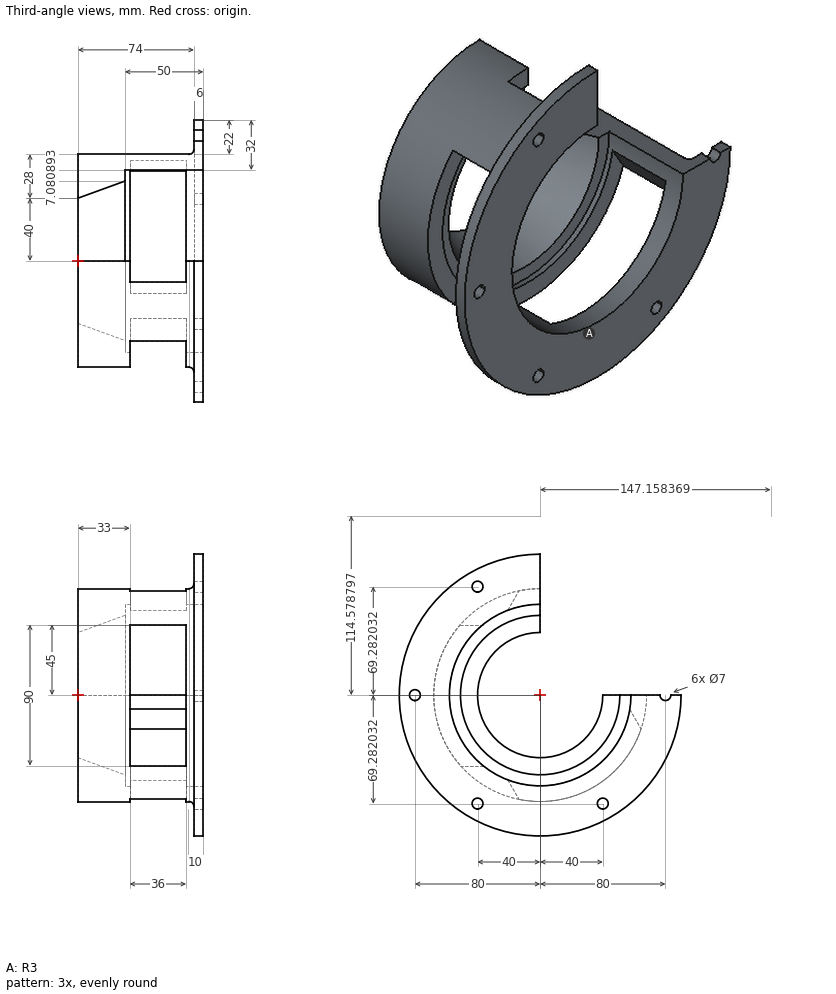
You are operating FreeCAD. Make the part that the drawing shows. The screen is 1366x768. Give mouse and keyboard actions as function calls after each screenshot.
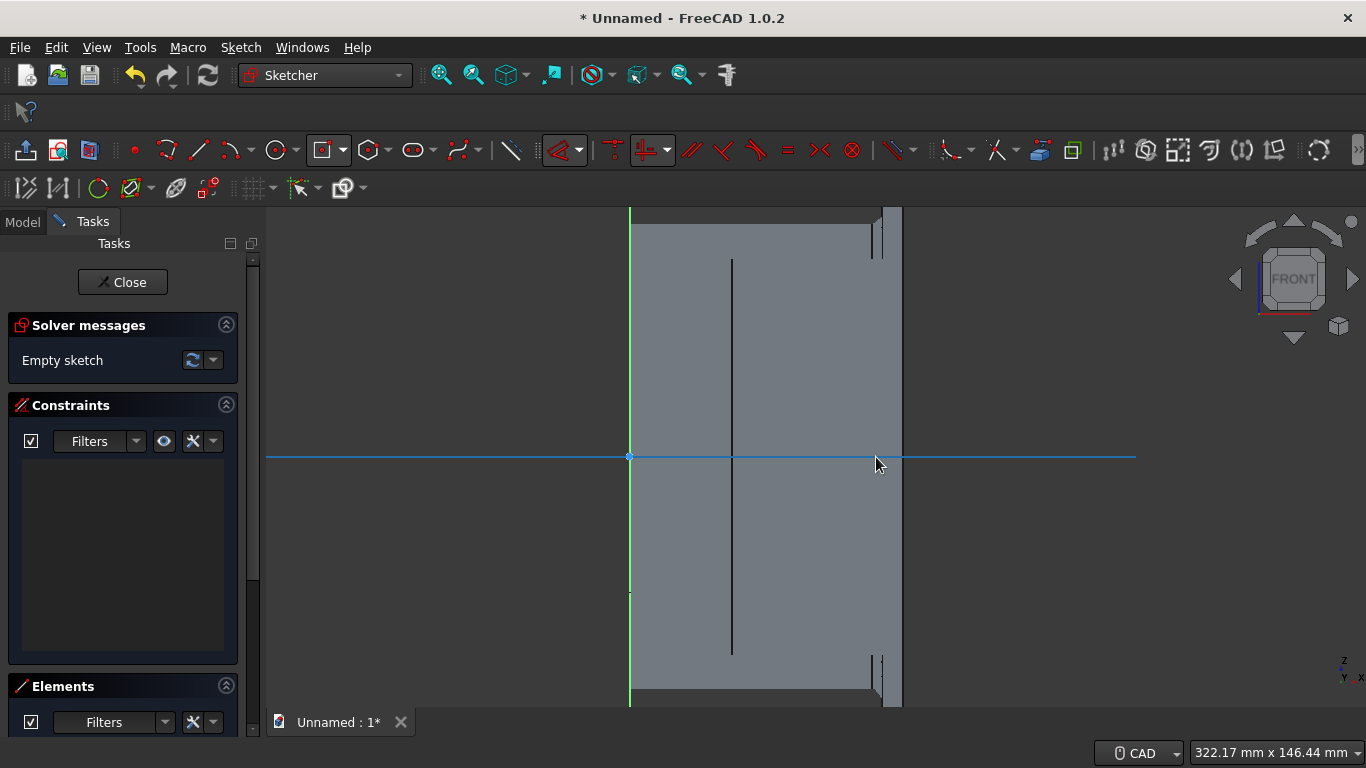
key(g)
key(r)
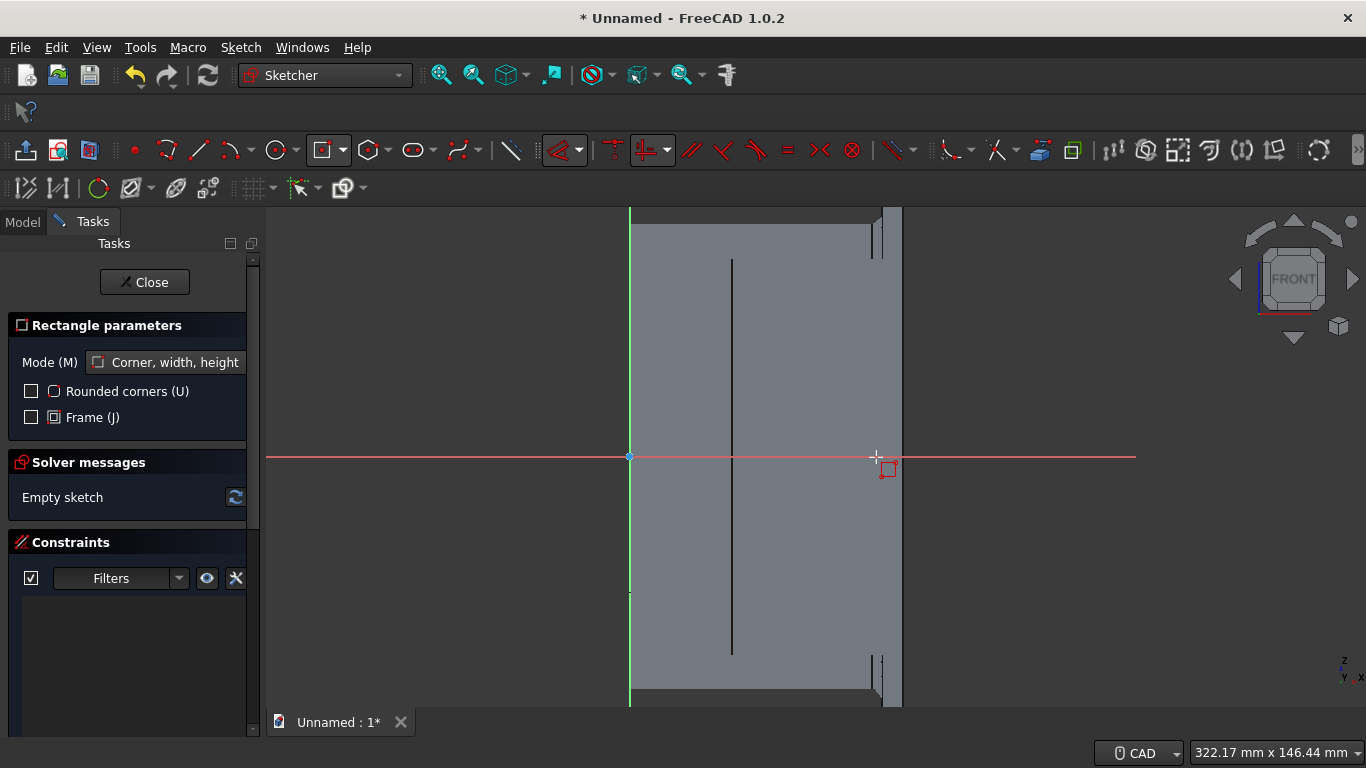
click(742, 303)
click(865, 610)
key(Escape)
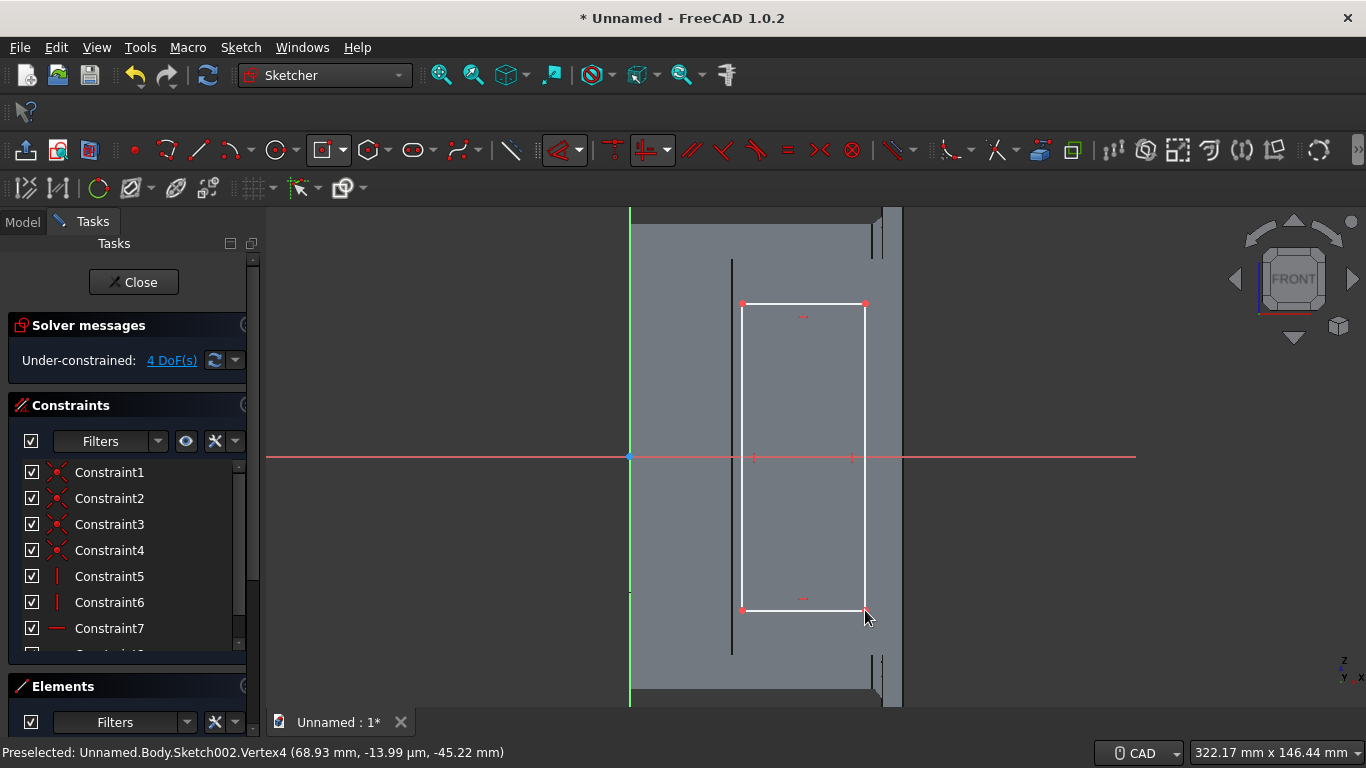
click(742, 396)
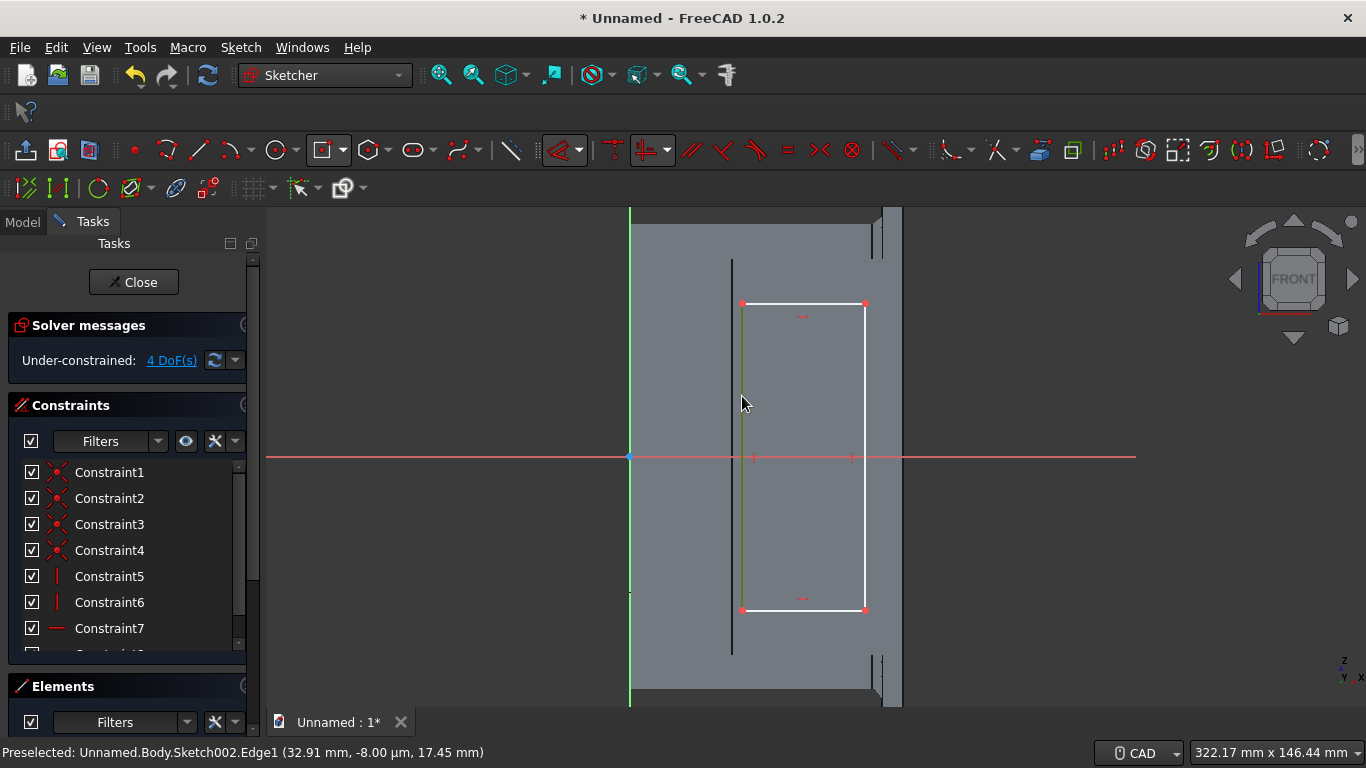
key(i)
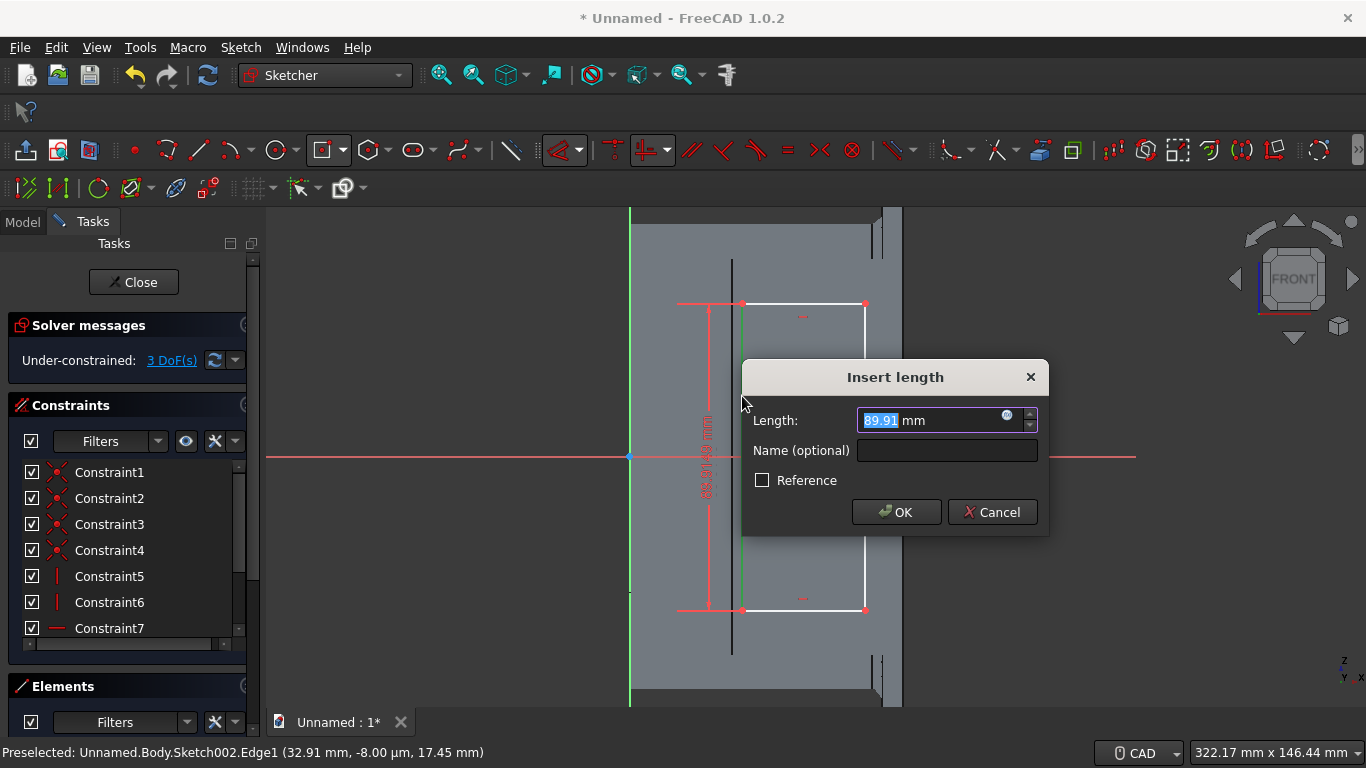
text(90)
key(Return)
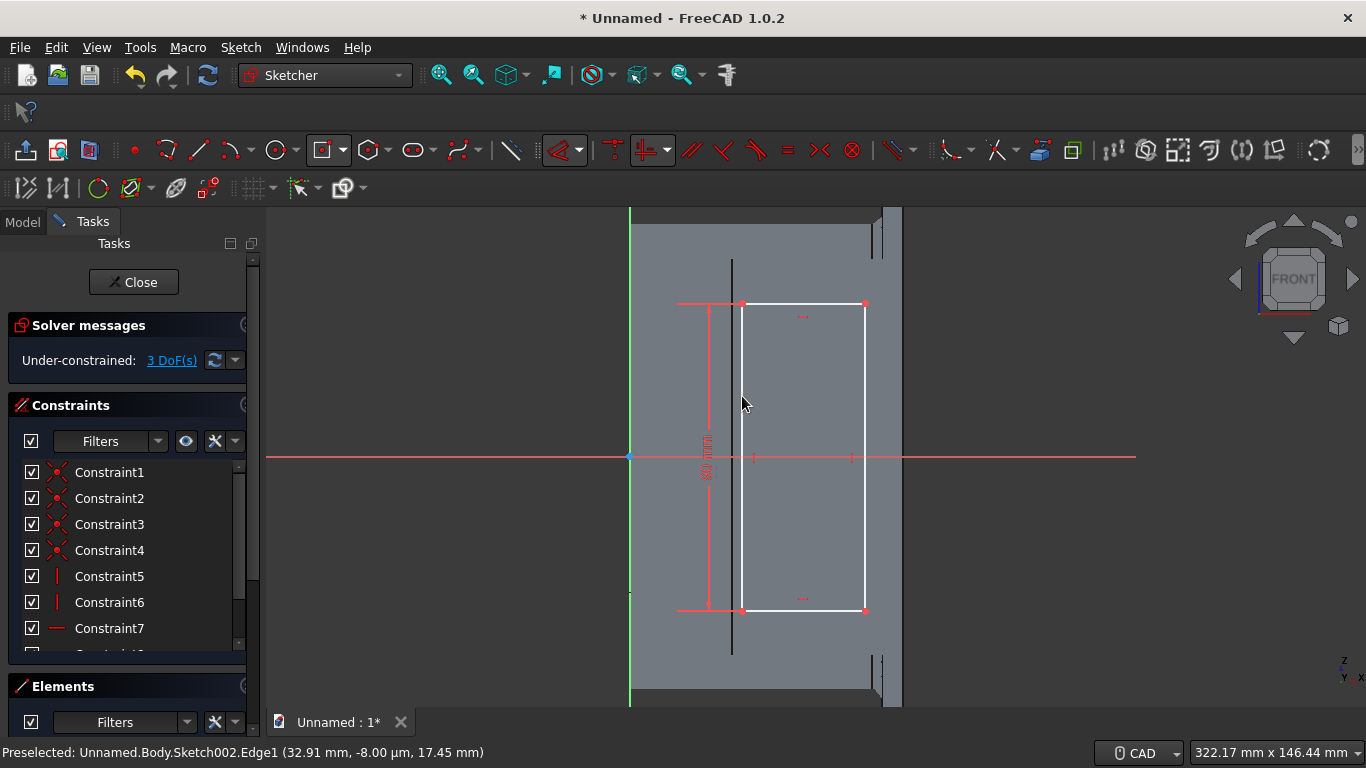
click(779, 611)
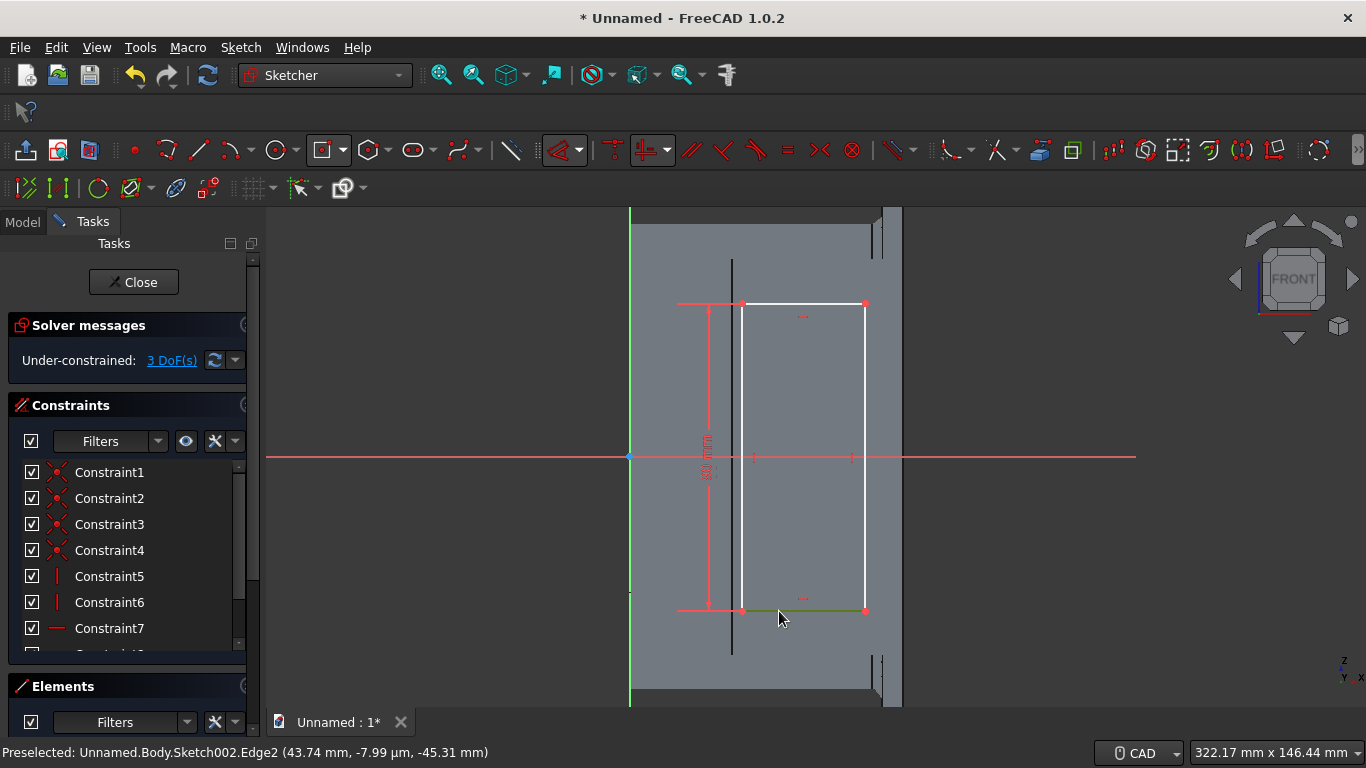
key(l)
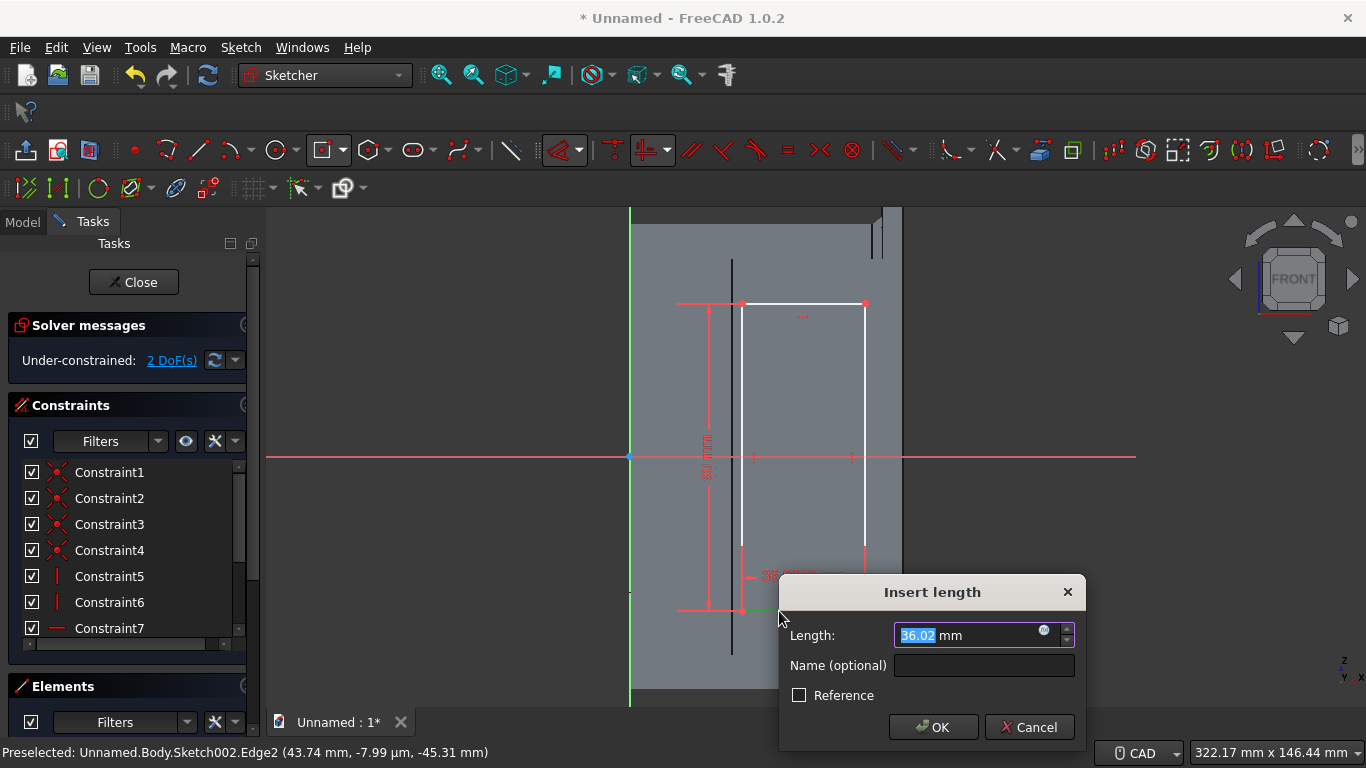
text(36)
key(Return)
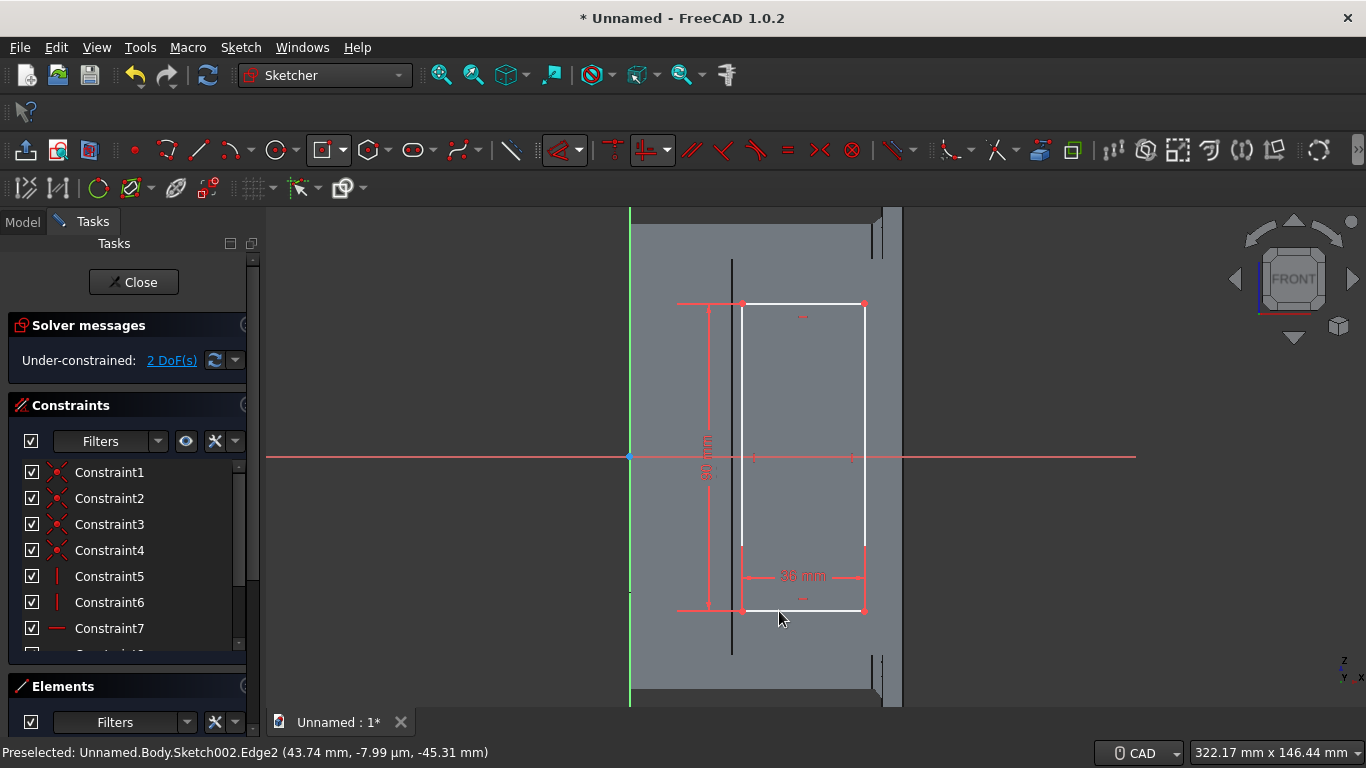
click(742, 304)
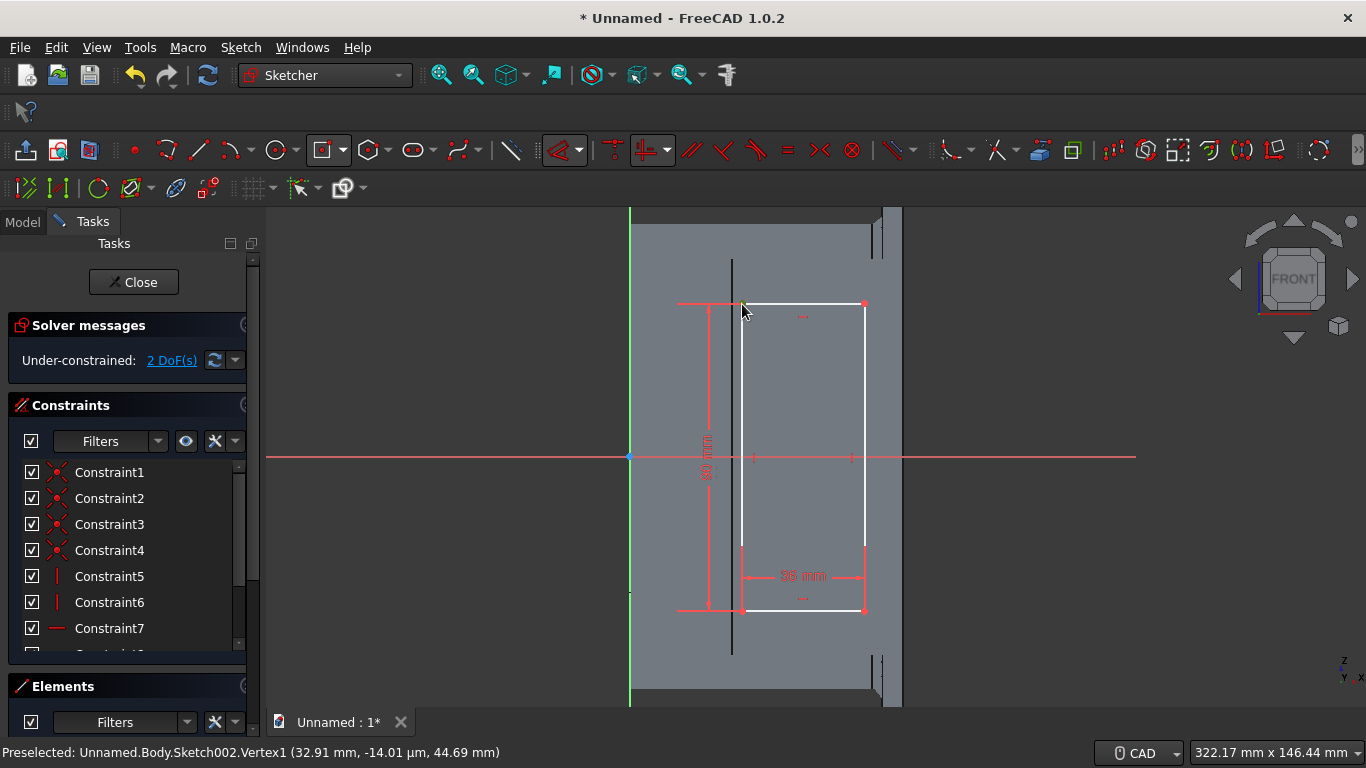
key(l)